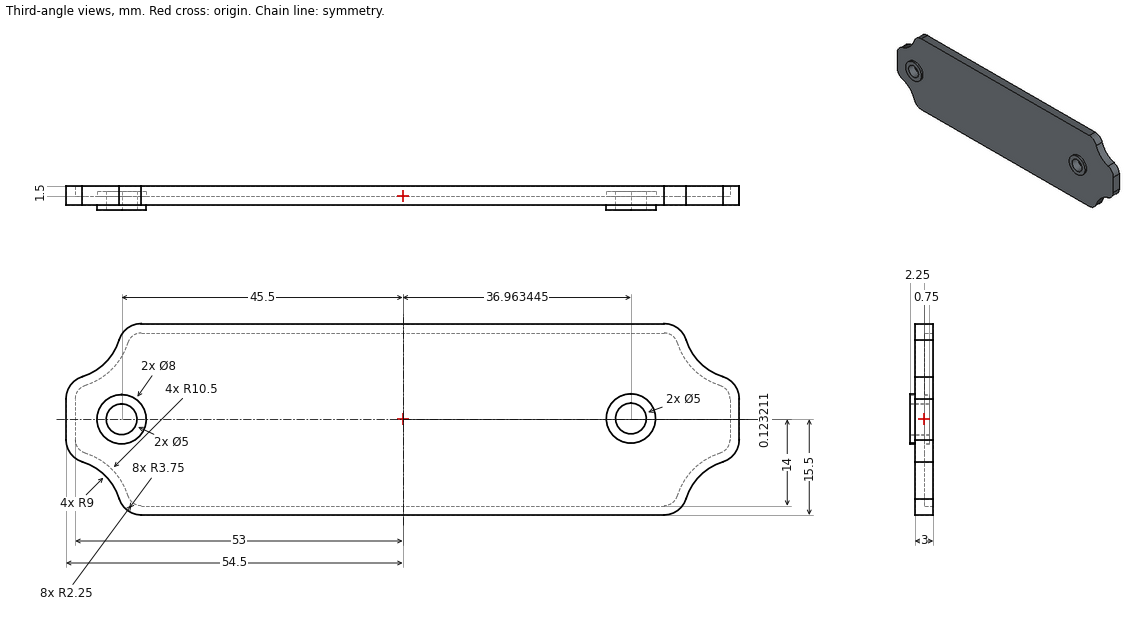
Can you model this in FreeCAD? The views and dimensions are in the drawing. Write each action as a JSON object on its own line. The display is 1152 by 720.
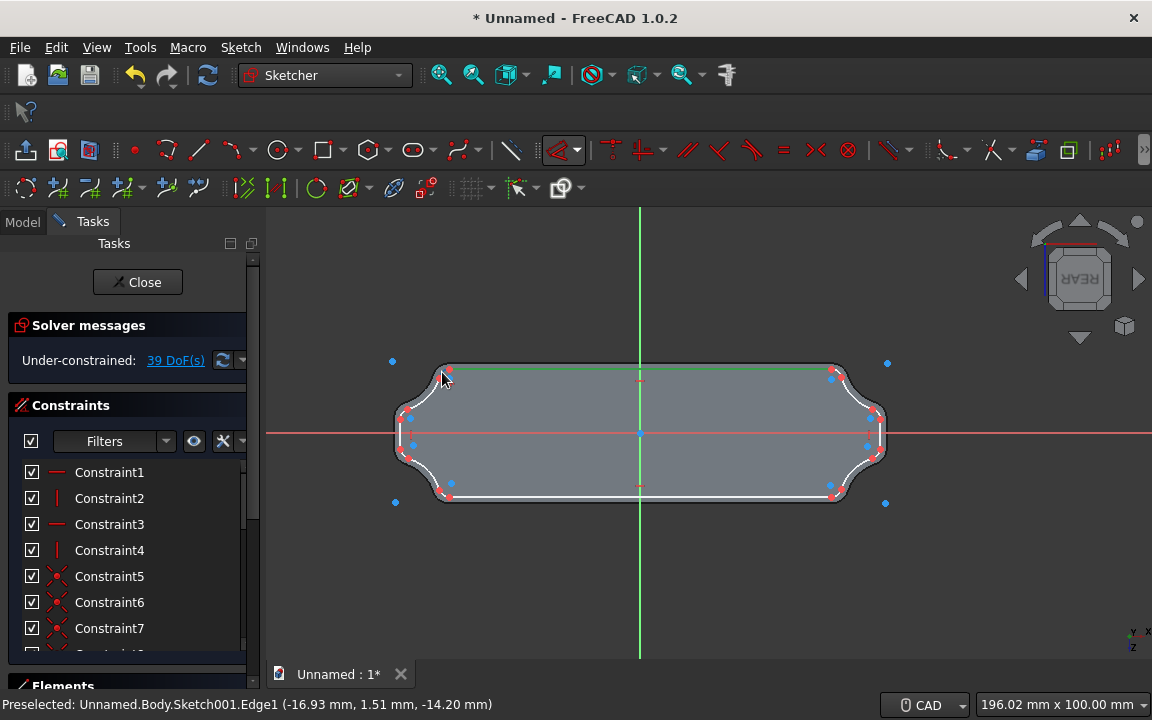
{"action": "scroll", "coordinate": [840, 374], "scroll_direction": "up", "scroll_amount": 6}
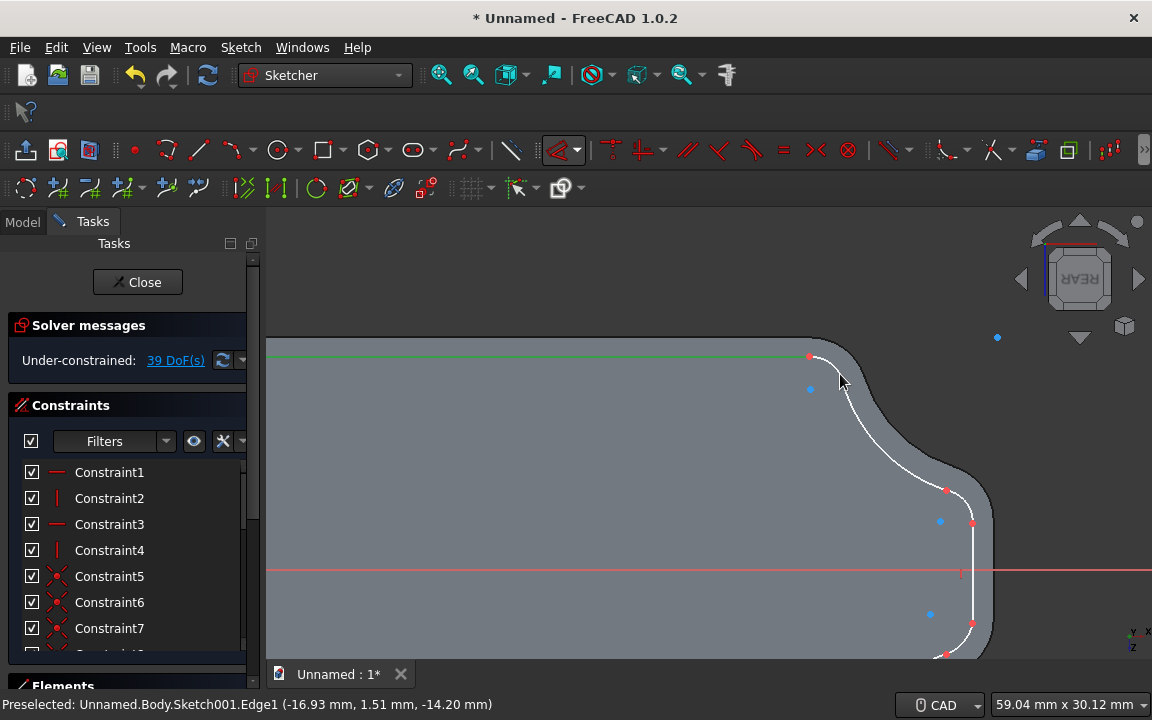
{"action": "left_click", "coordinate": [838, 372]}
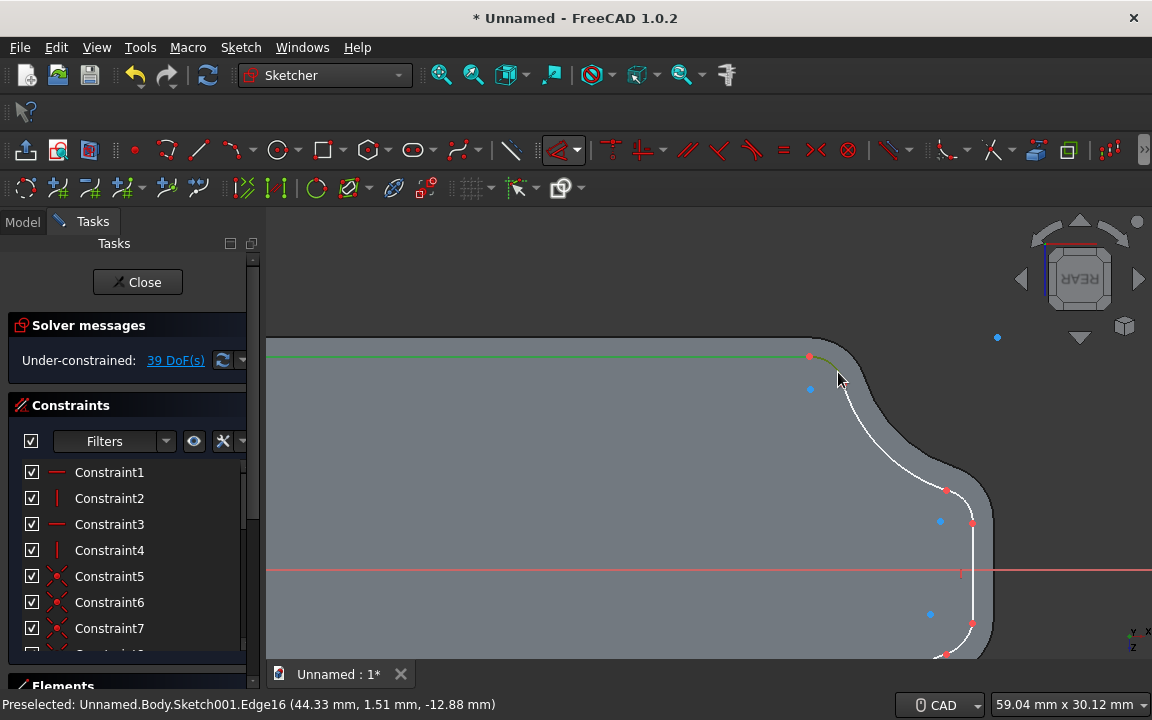
{"action": "left_click", "coordinate": [752, 150]}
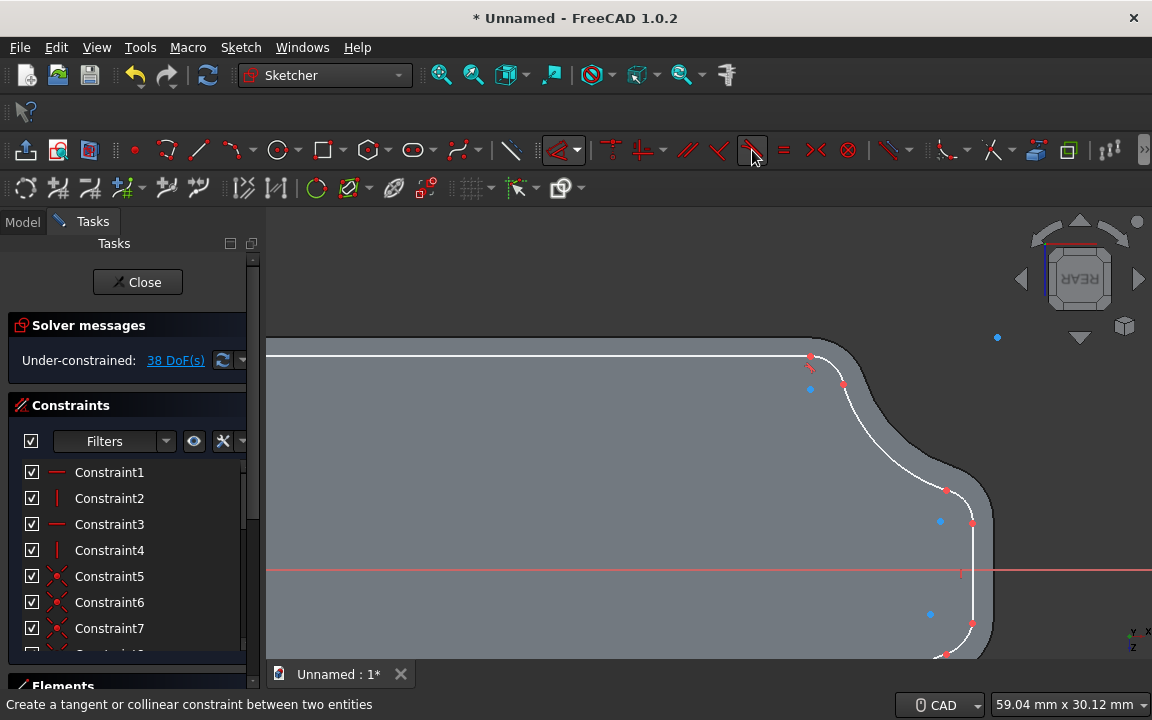
{"action": "scroll", "coordinate": [841, 374], "scroll_direction": "down", "scroll_amount": 6}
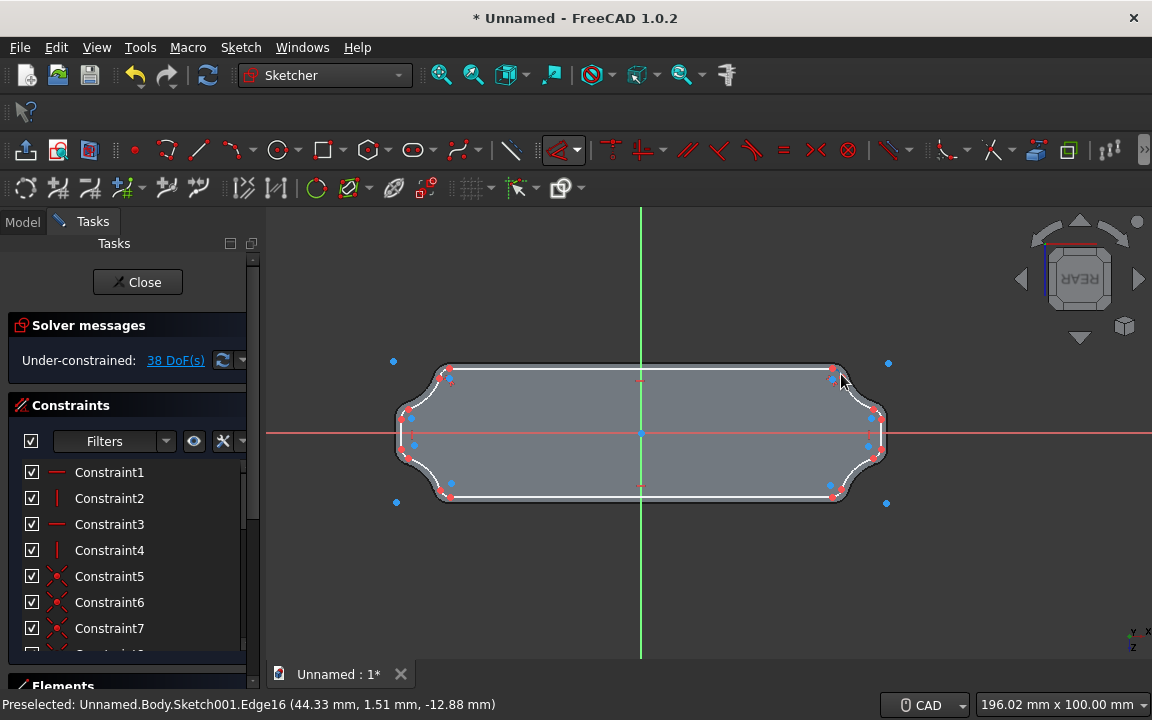
{"action": "scroll", "coordinate": [401, 428], "scroll_direction": "up", "scroll_amount": 6}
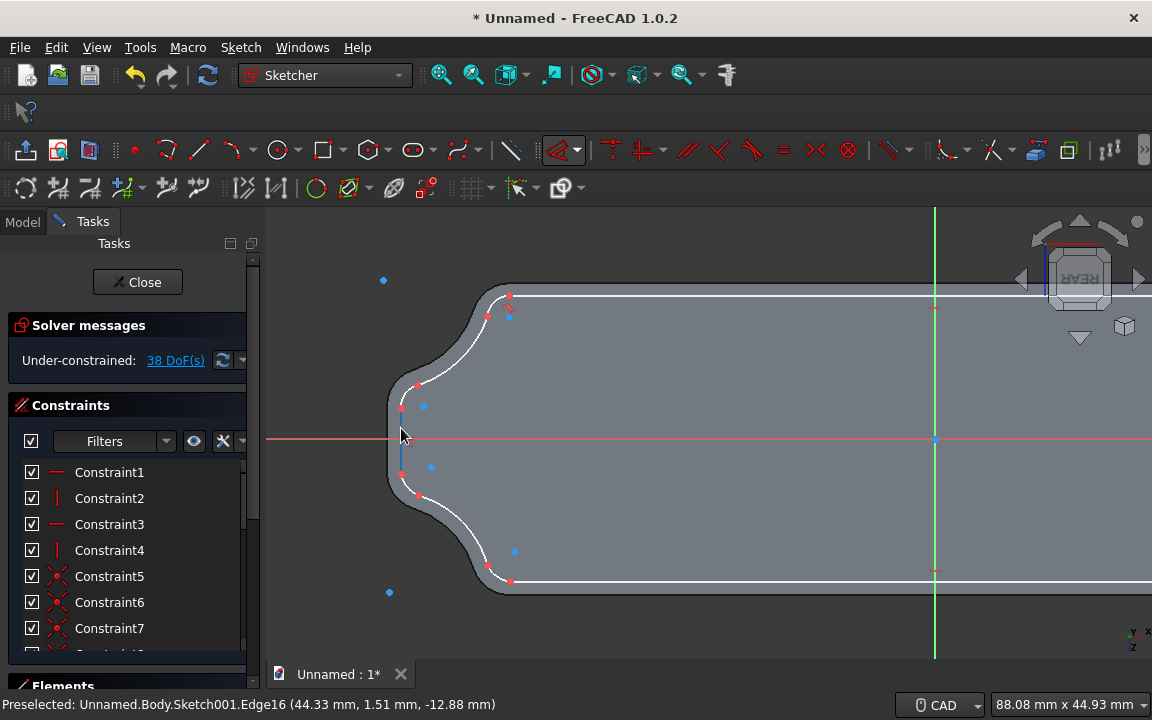
{"action": "left_click", "coordinate": [401, 428]}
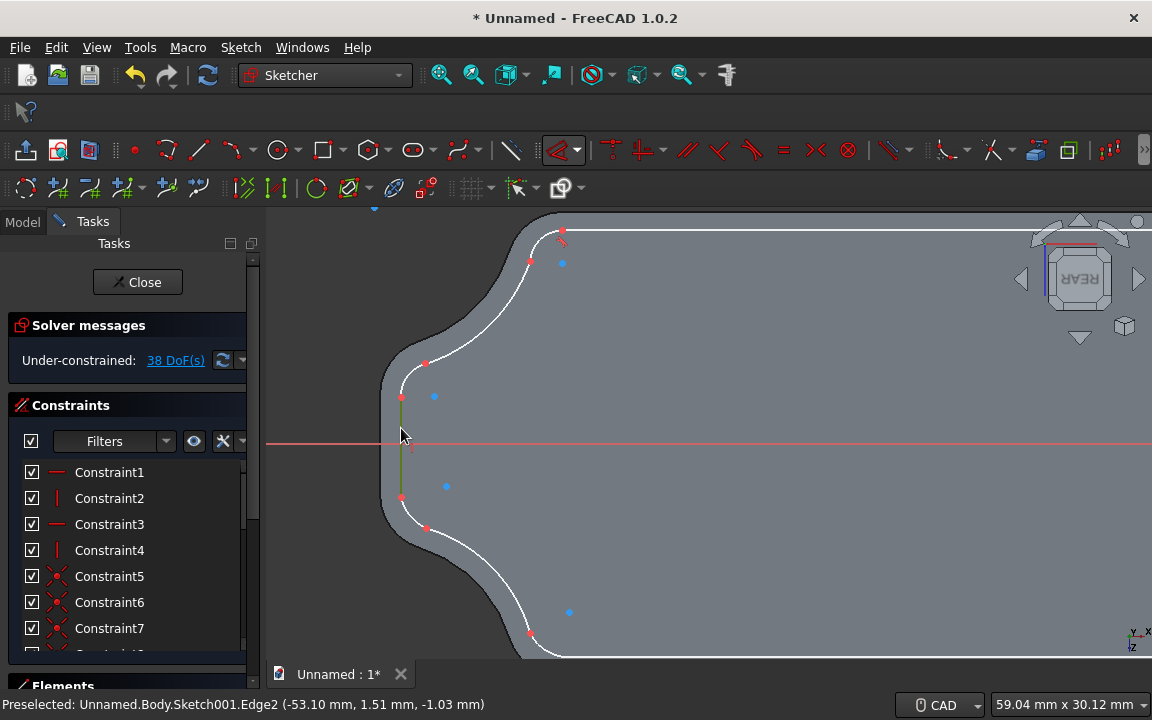
{"action": "left_click", "coordinate": [414, 370]}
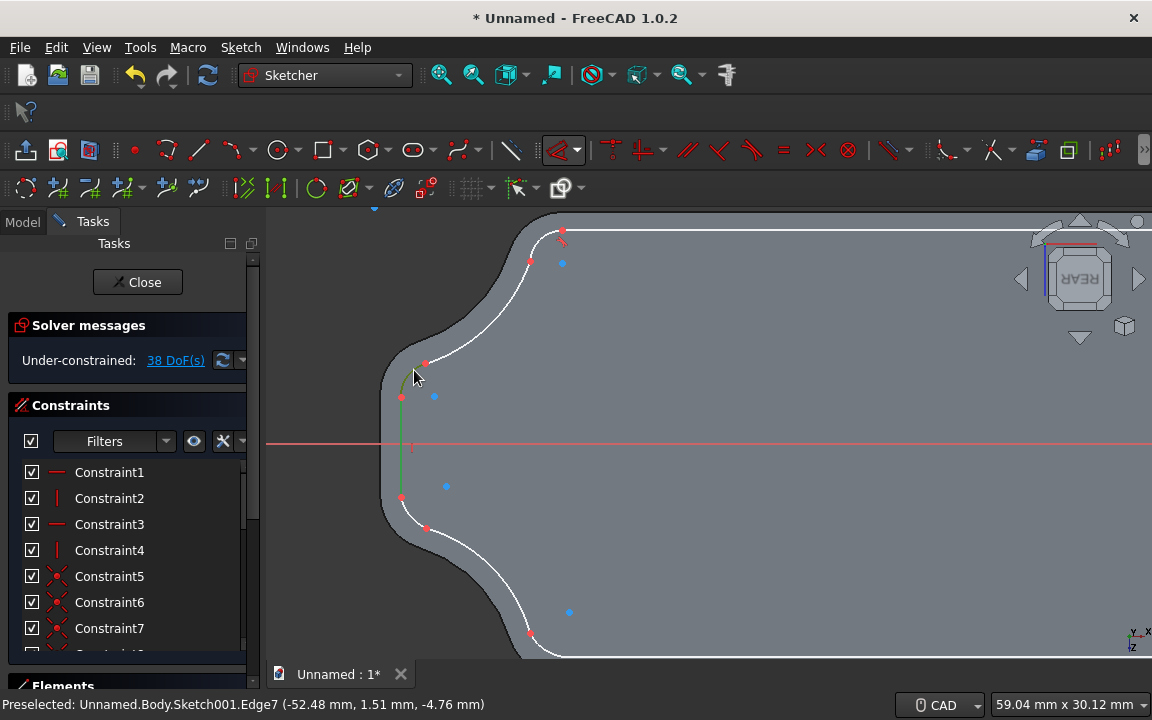
{"action": "left_click", "coordinate": [752, 150]}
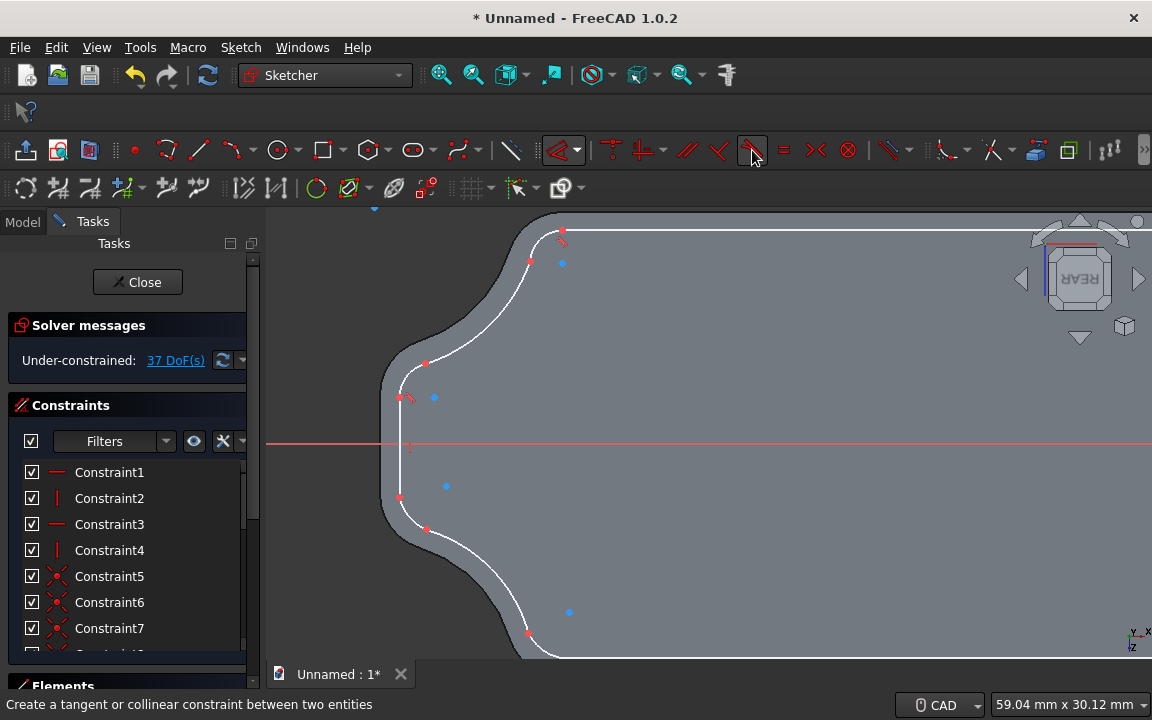
{"action": "left_click", "coordinate": [400, 428]}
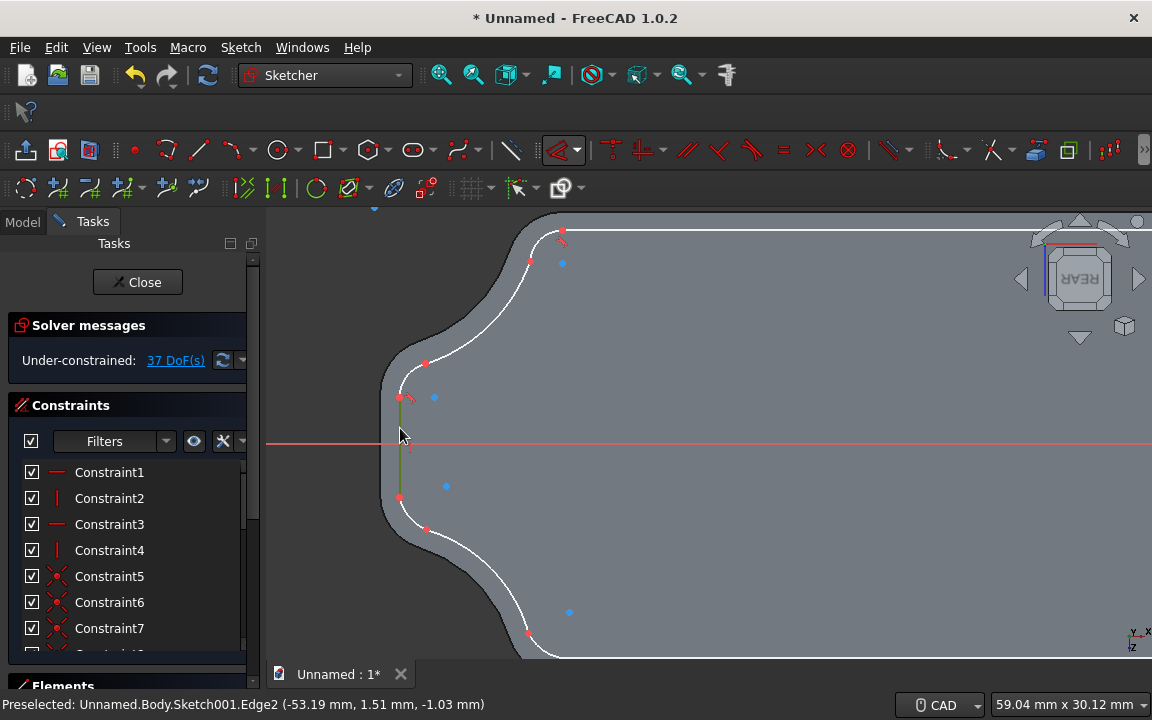
{"action": "left_click", "coordinate": [404, 510]}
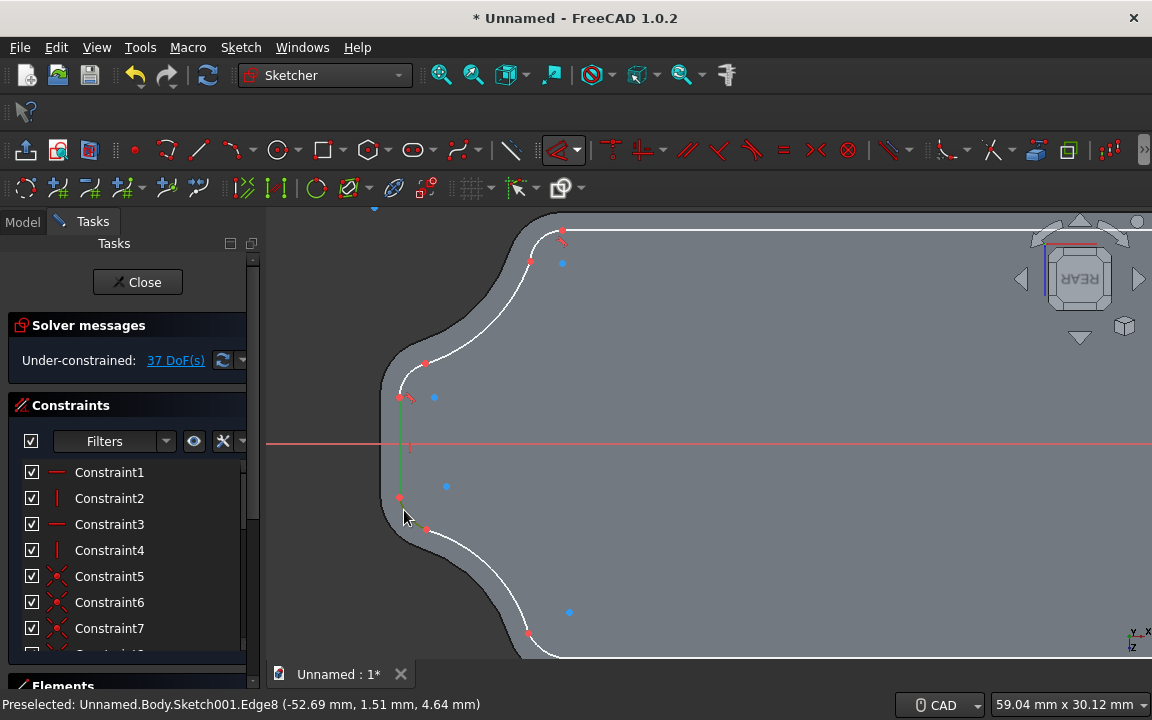
{"action": "left_click", "coordinate": [752, 150]}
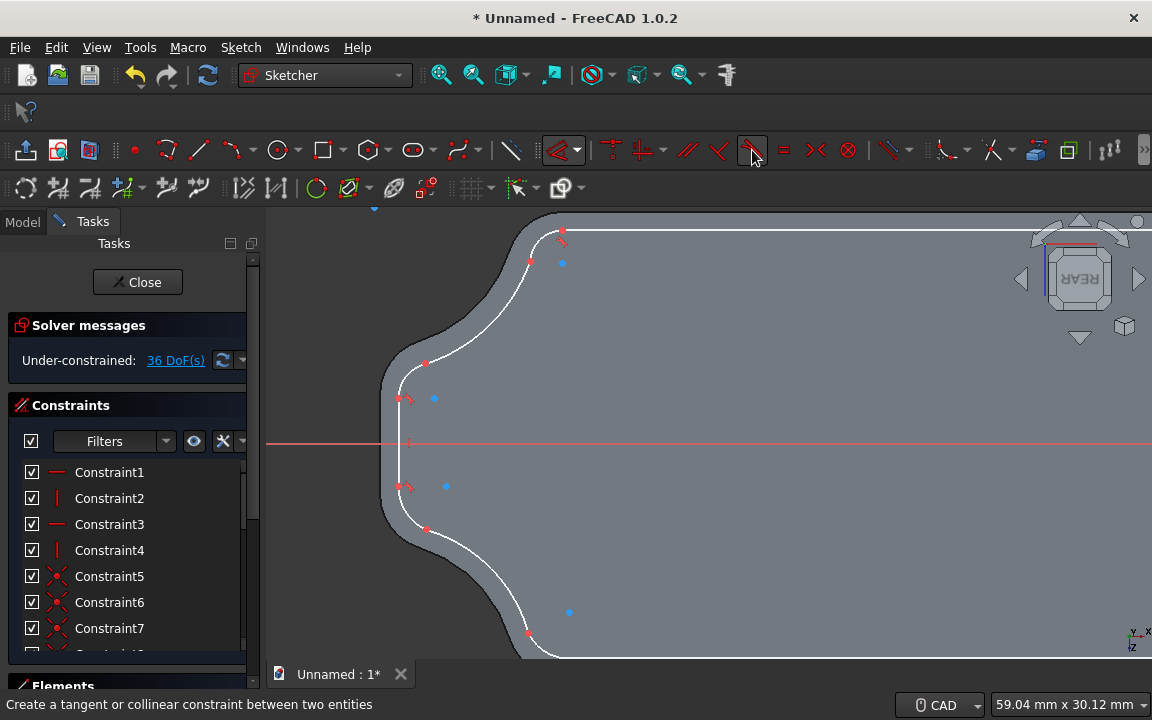
{"action": "scroll", "coordinate": [400, 428], "scroll_direction": "down", "scroll_amount": 6}